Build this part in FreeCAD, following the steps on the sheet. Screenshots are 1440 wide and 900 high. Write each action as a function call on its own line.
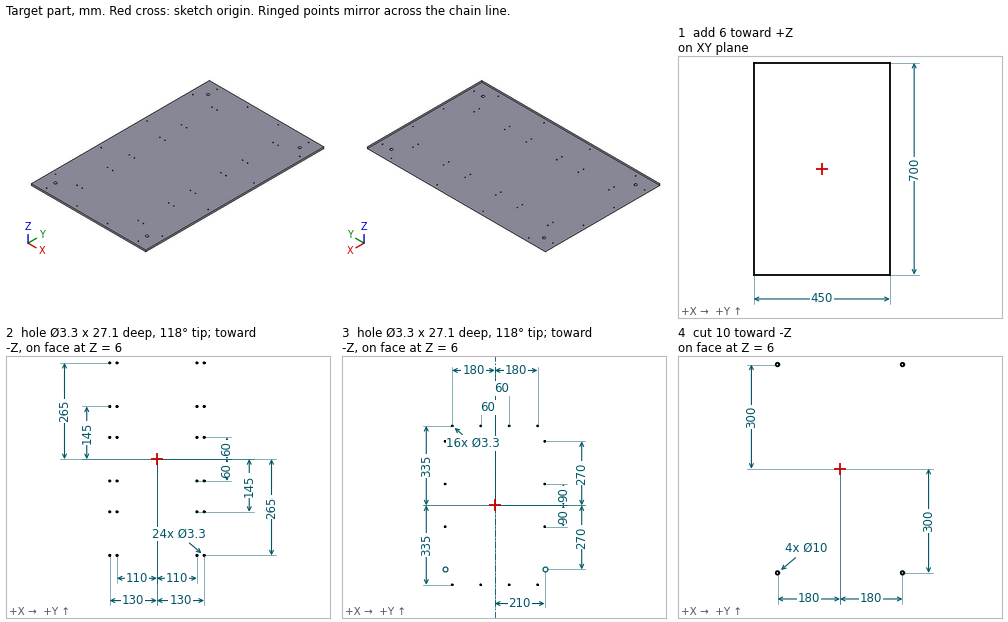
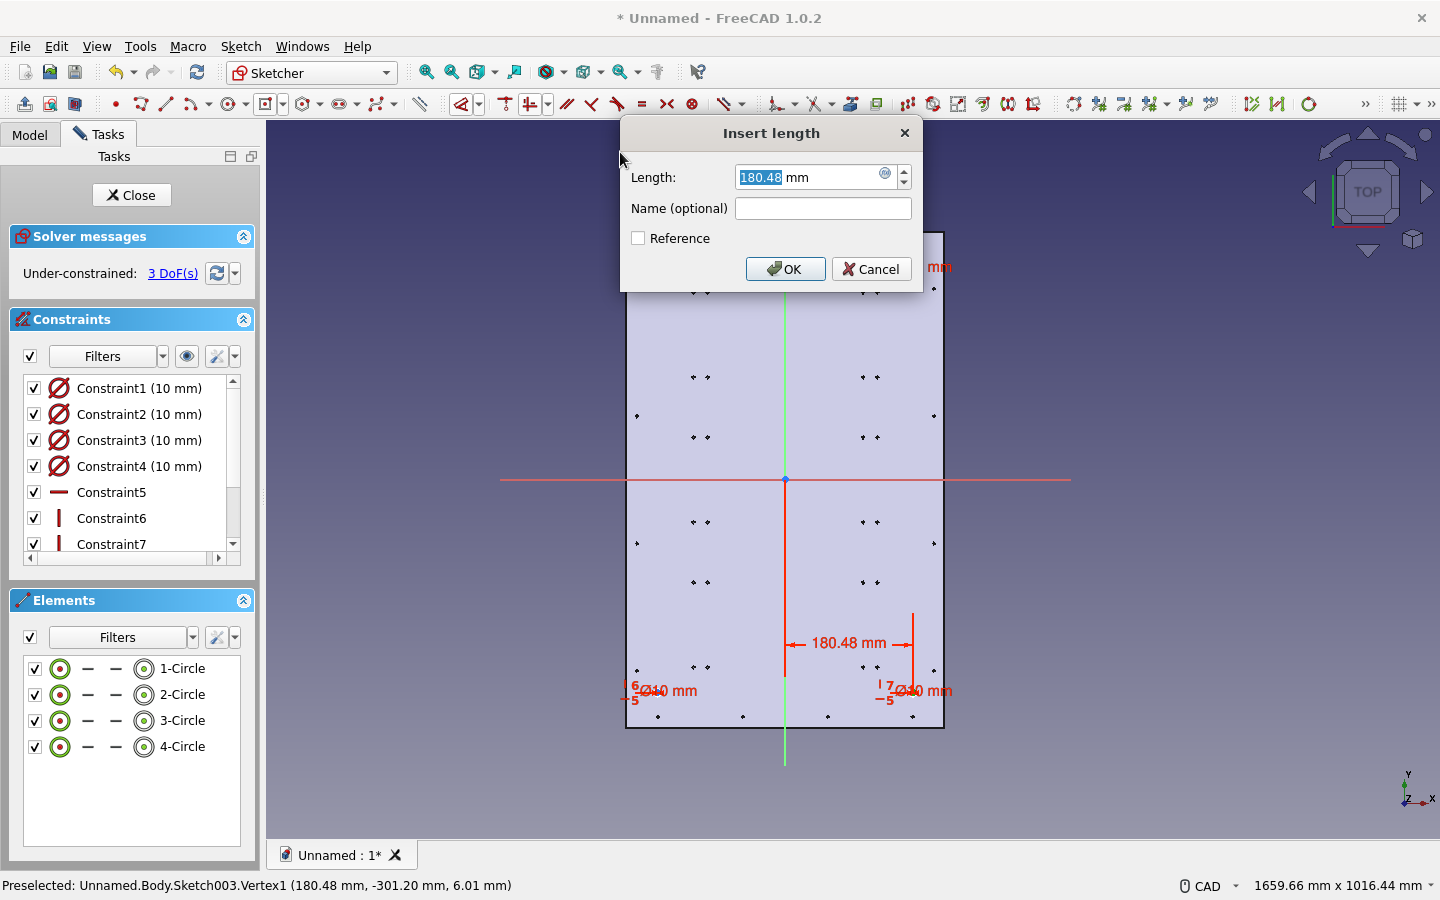
text(180)
key(Return)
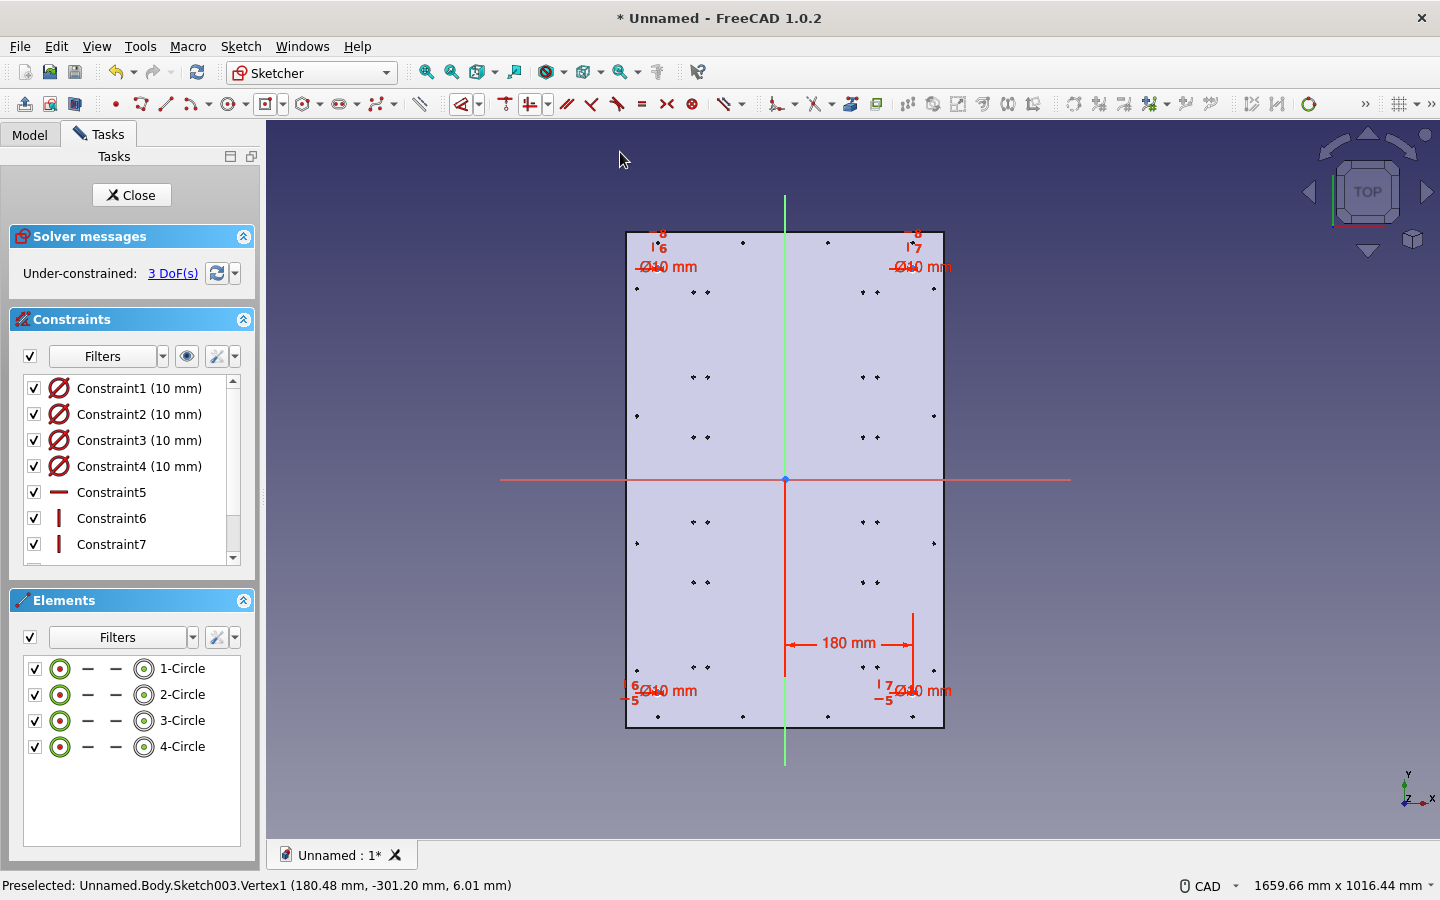
click(913, 693)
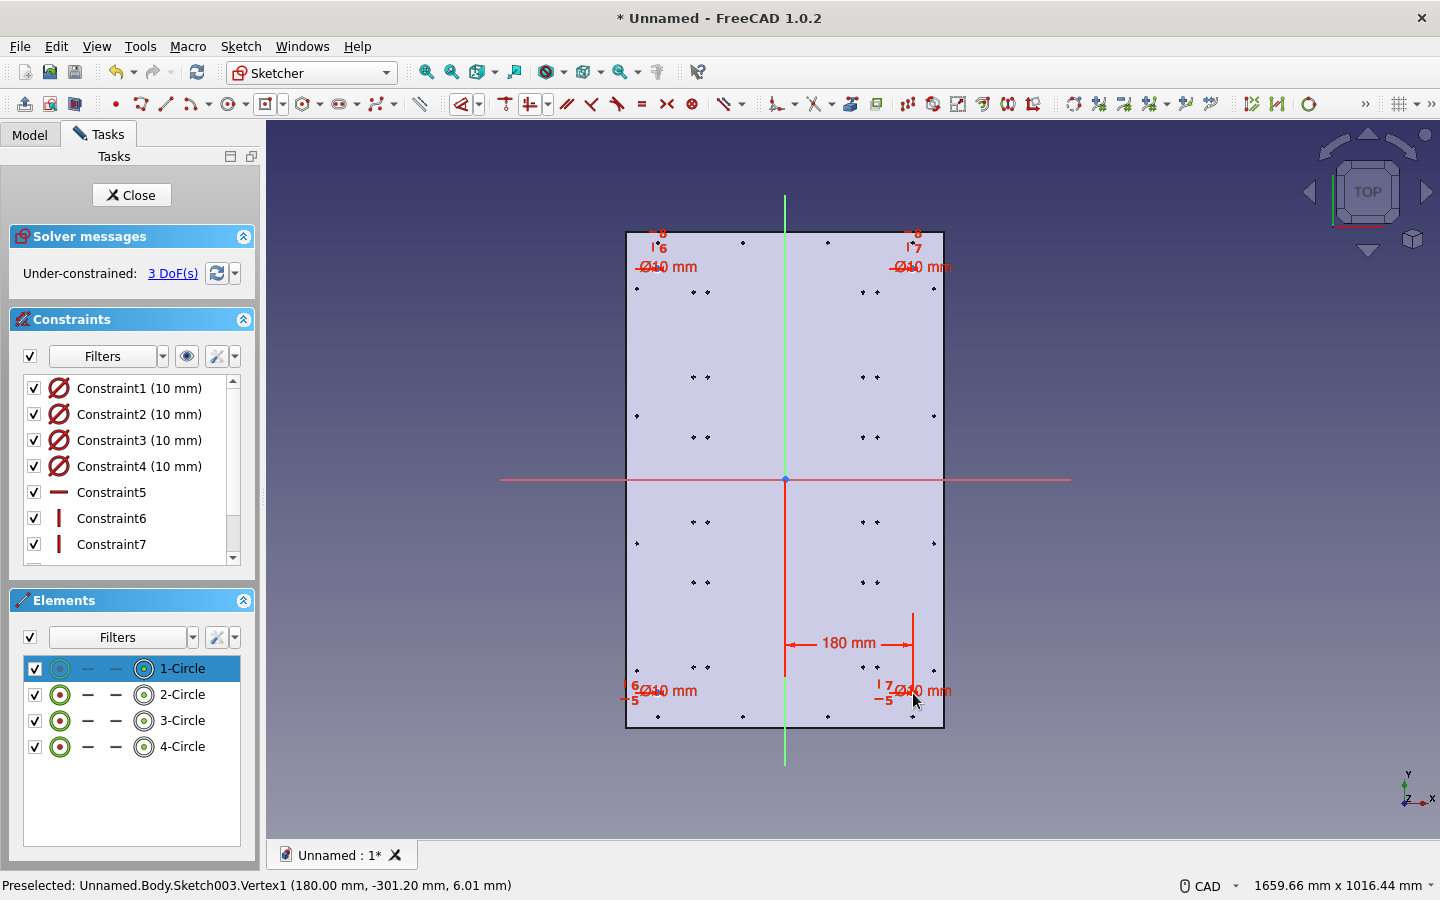
click(478, 104)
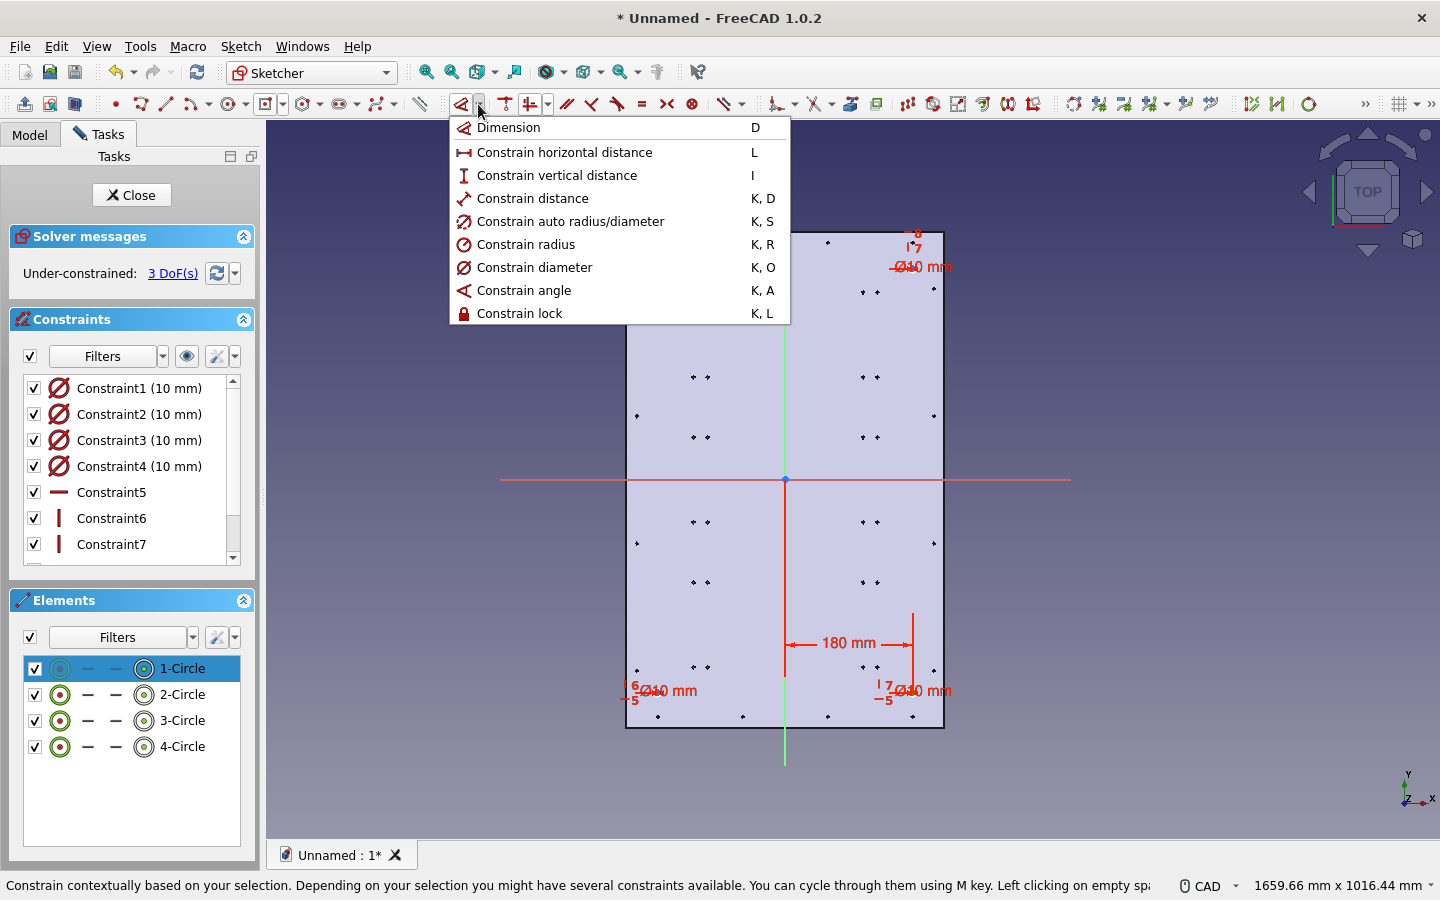
click(620, 176)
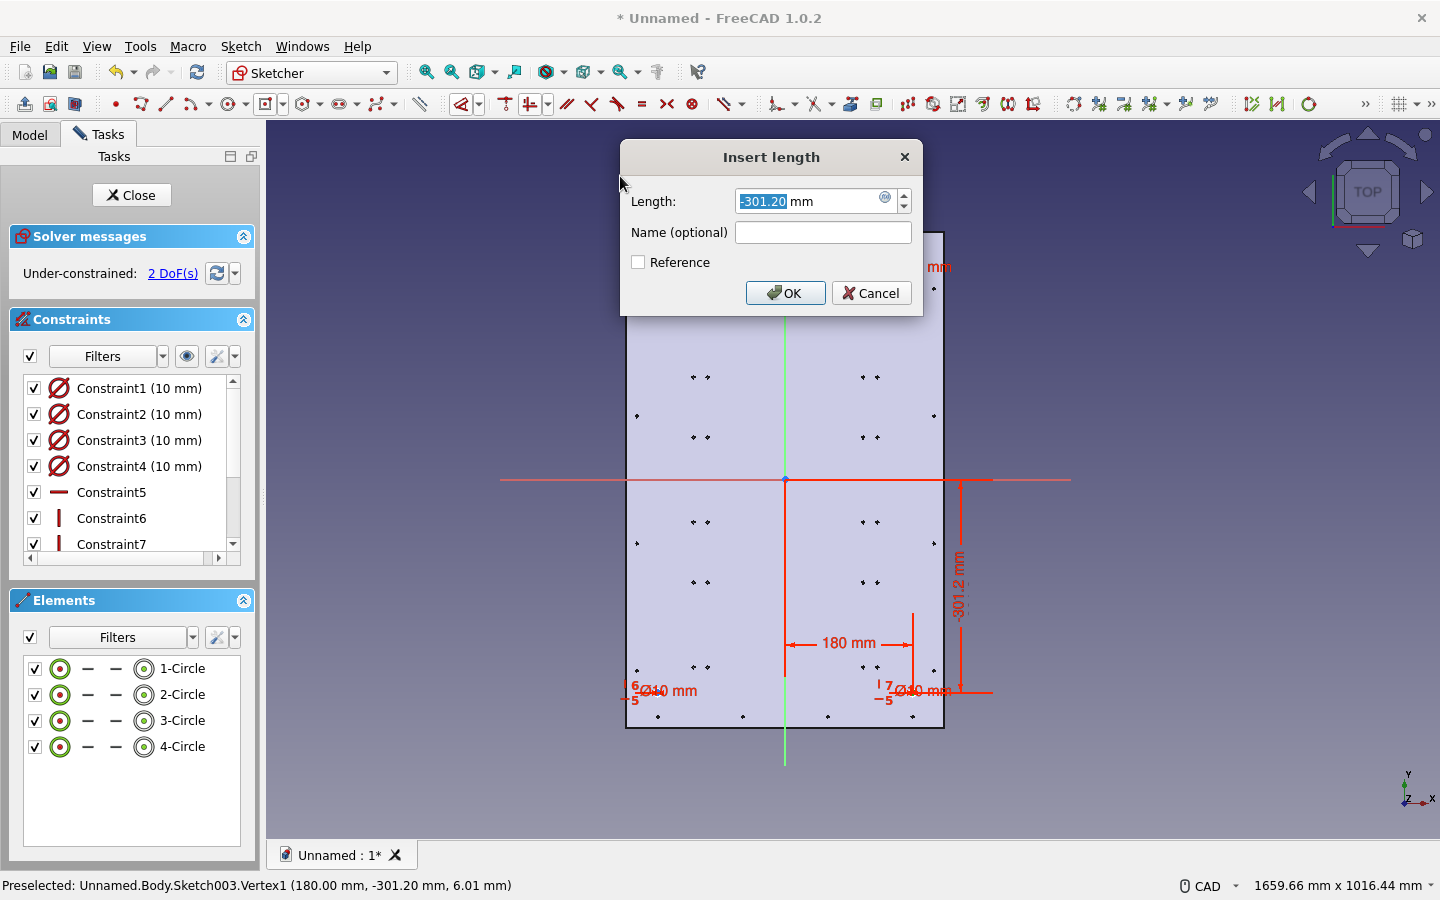
text(-300)
key(Return)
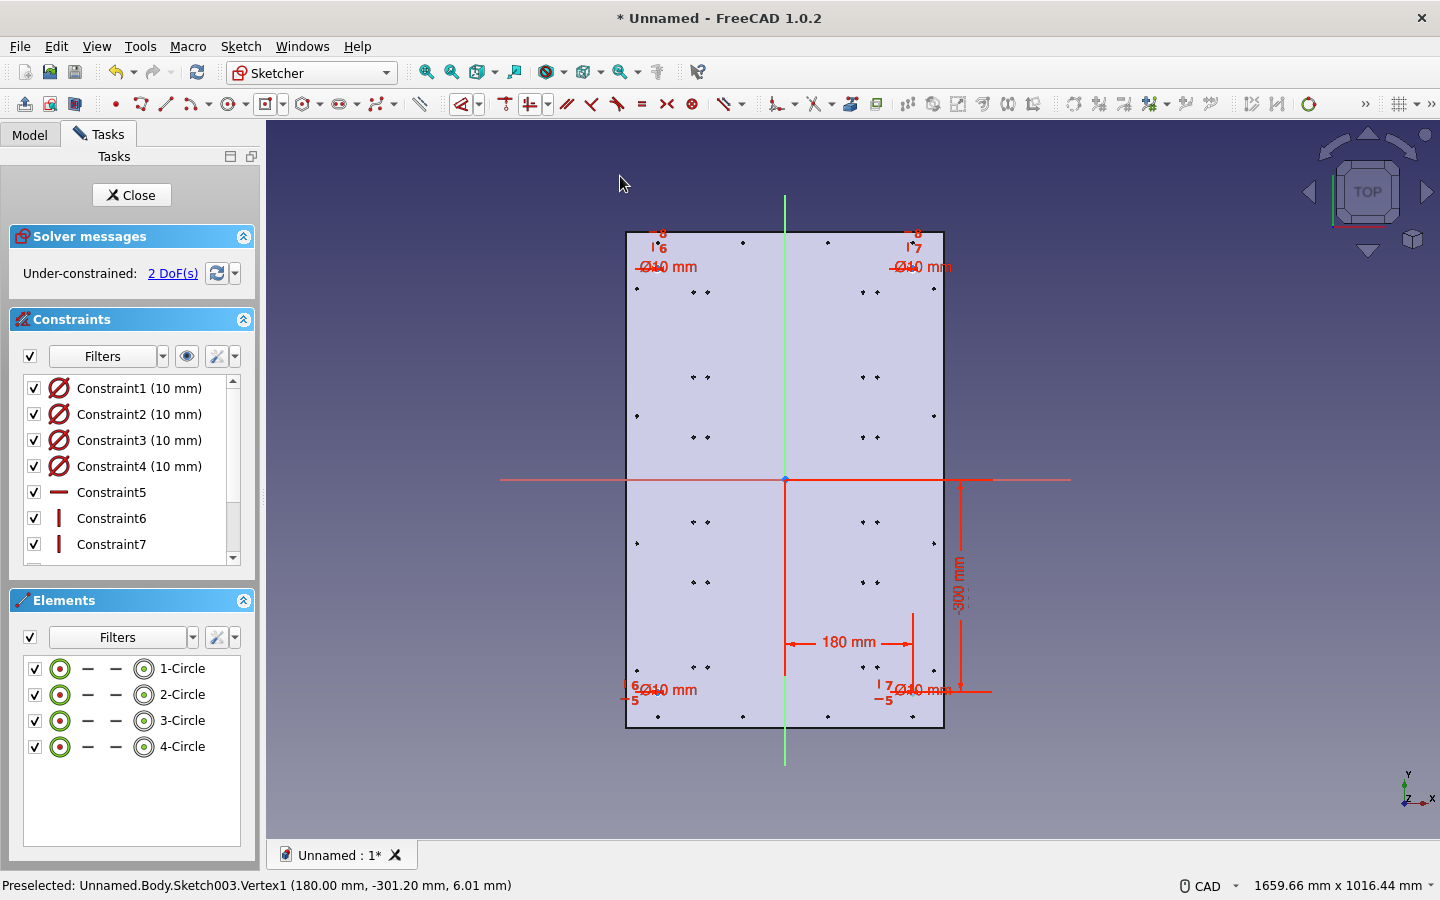
click(658, 692)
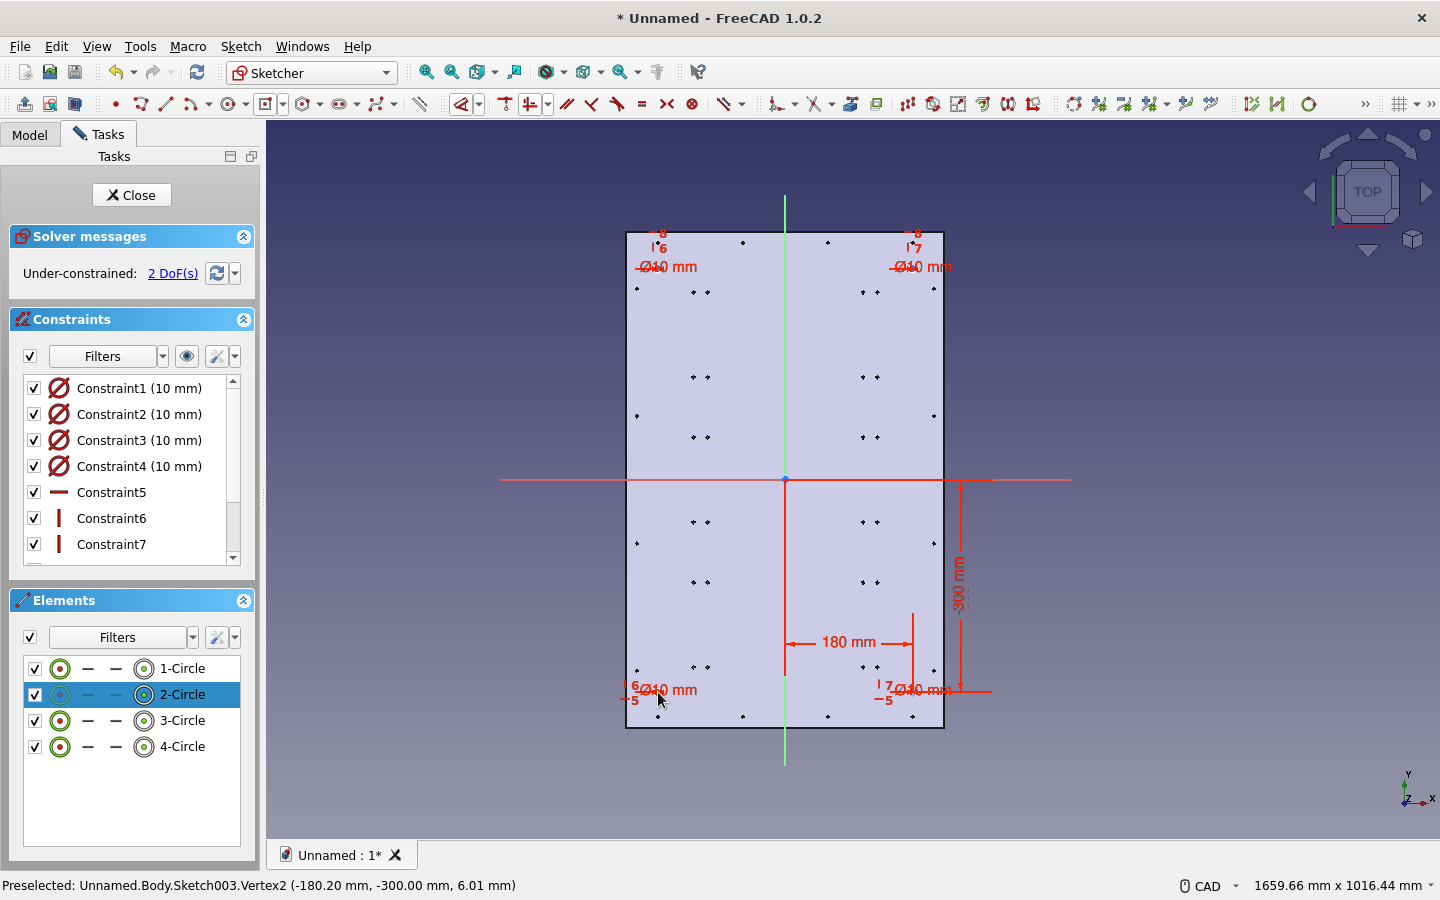
key(l)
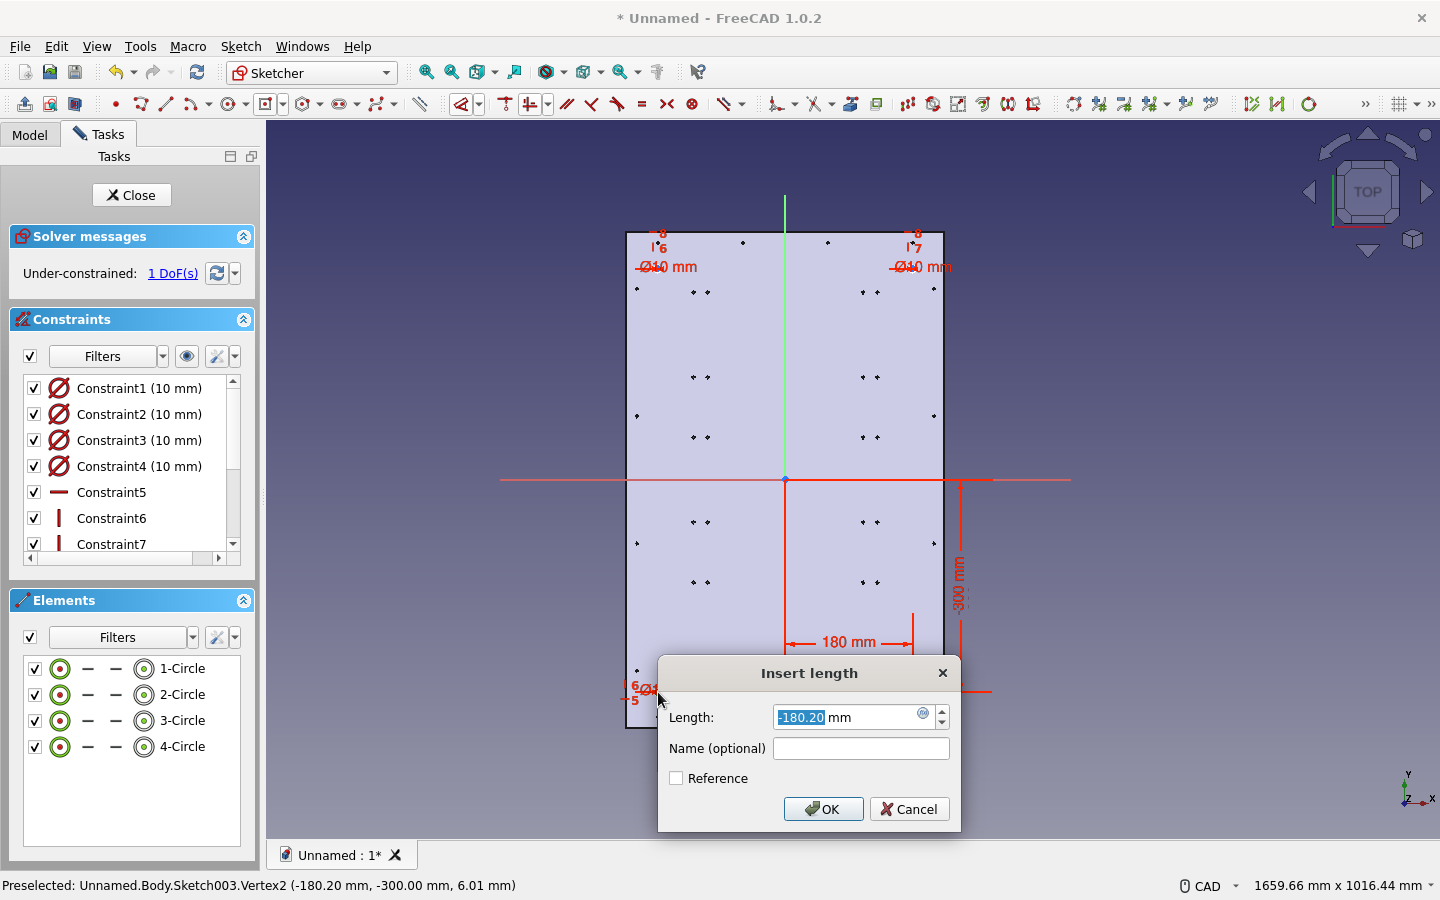
text(-180)
key(Return)